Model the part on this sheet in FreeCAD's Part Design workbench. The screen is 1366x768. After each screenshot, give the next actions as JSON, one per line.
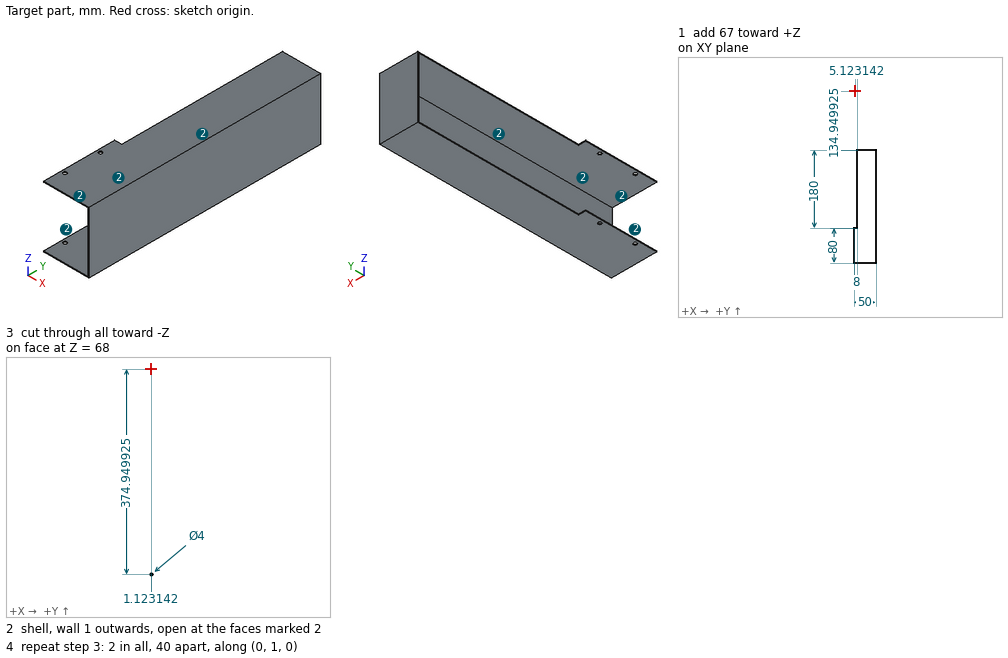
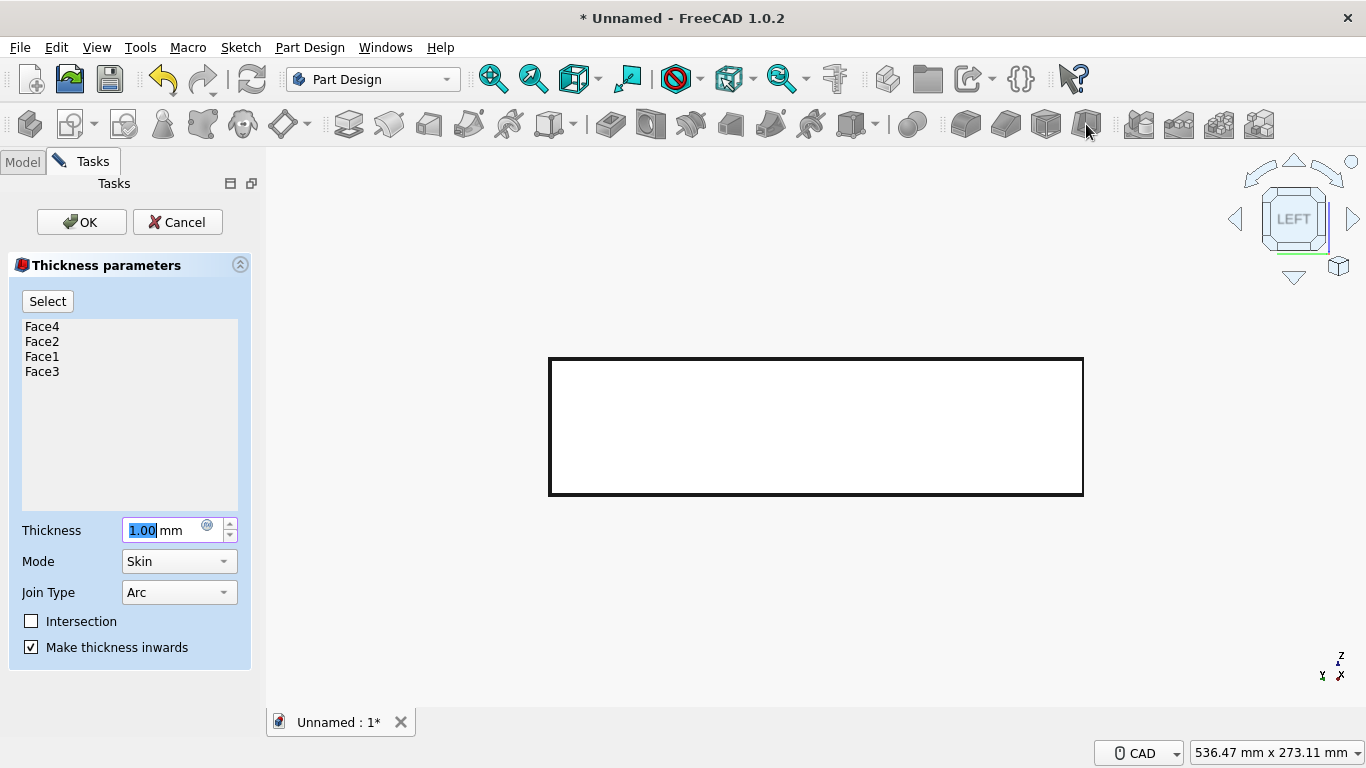
{"action": "type", "text": "1"}
{"action": "key", "text": "Tab"}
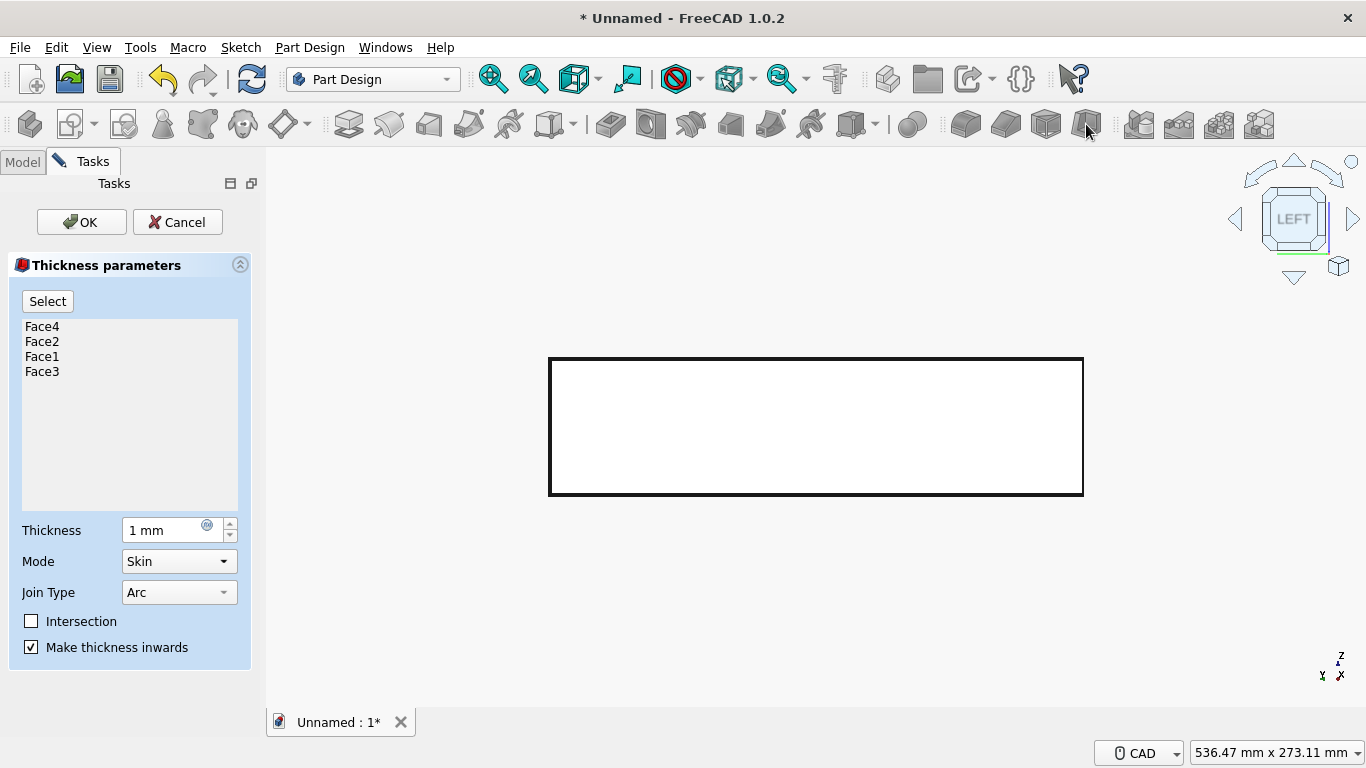
{"action": "left_click", "coordinate": [180, 592]}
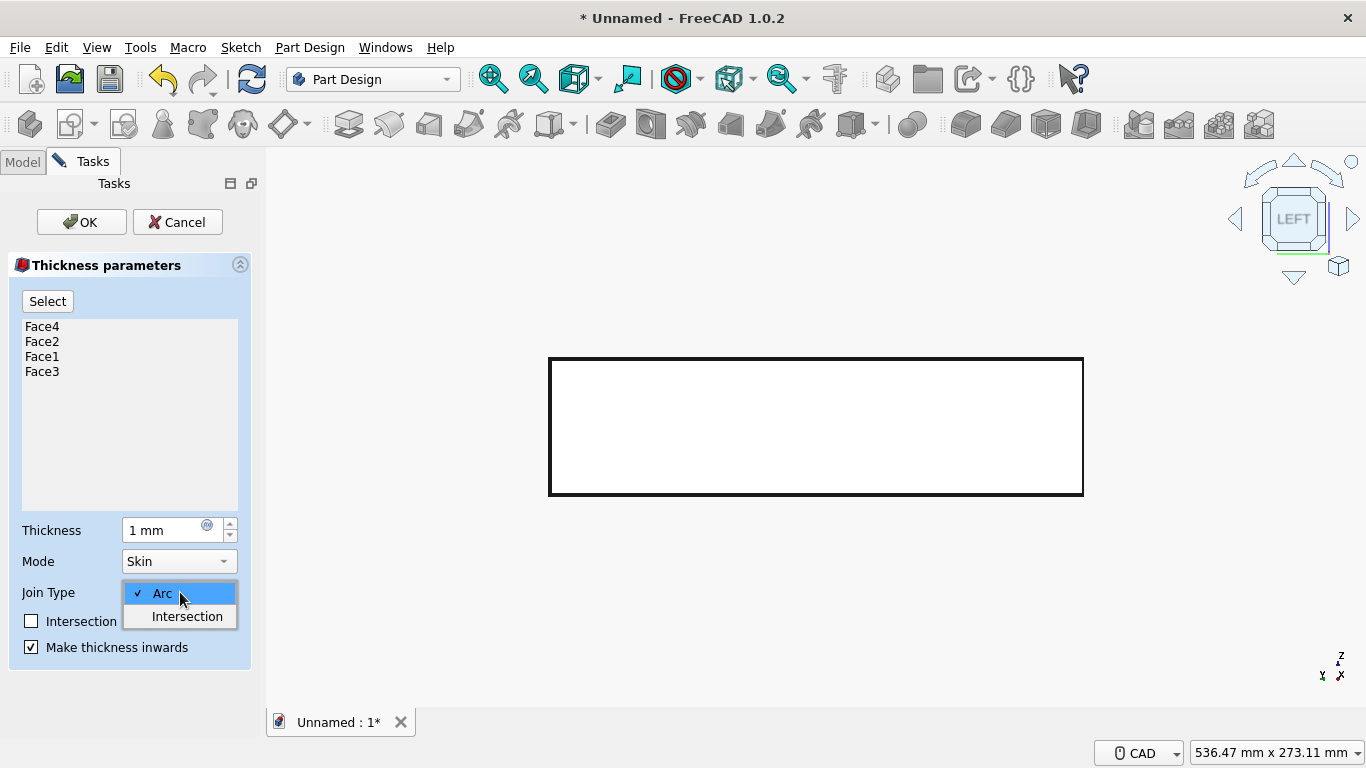
{"action": "left_click", "coordinate": [179, 616]}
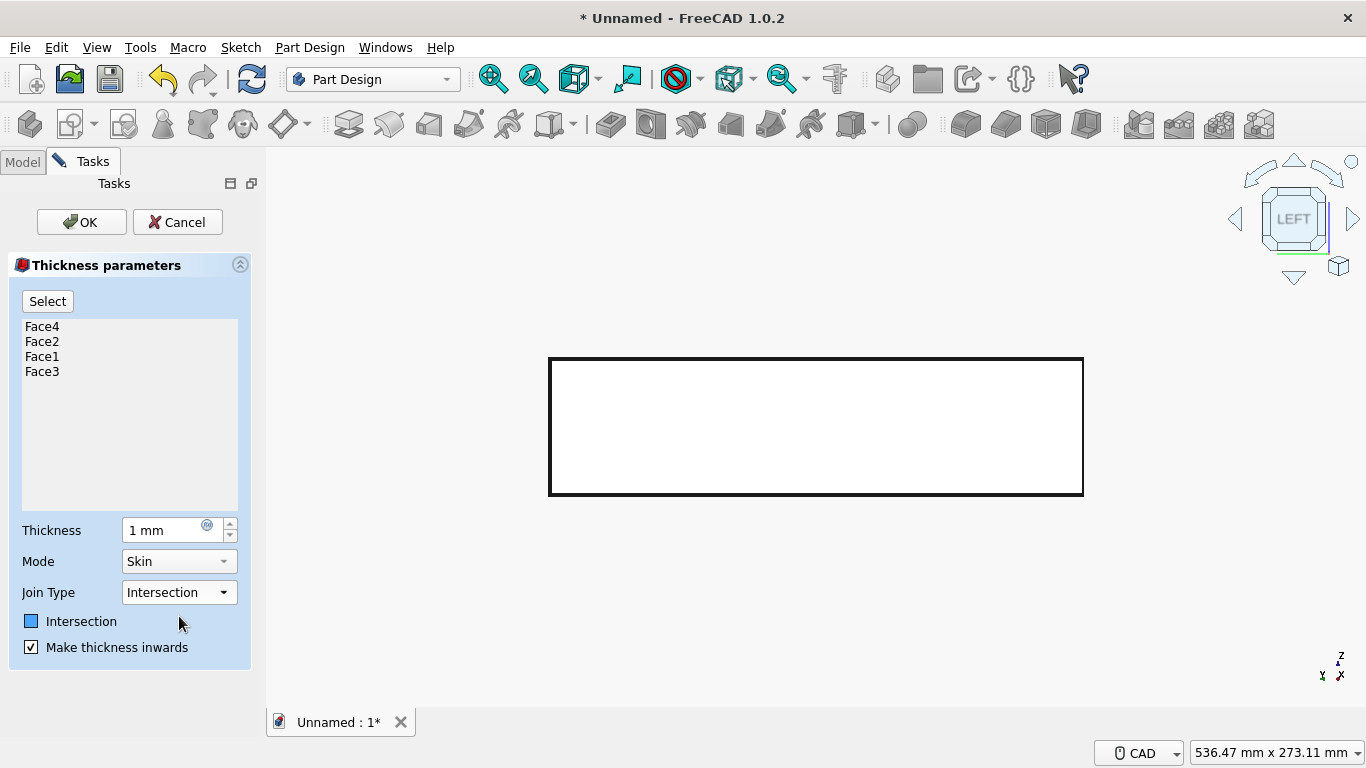
{"action": "left_click", "coordinate": [30, 647]}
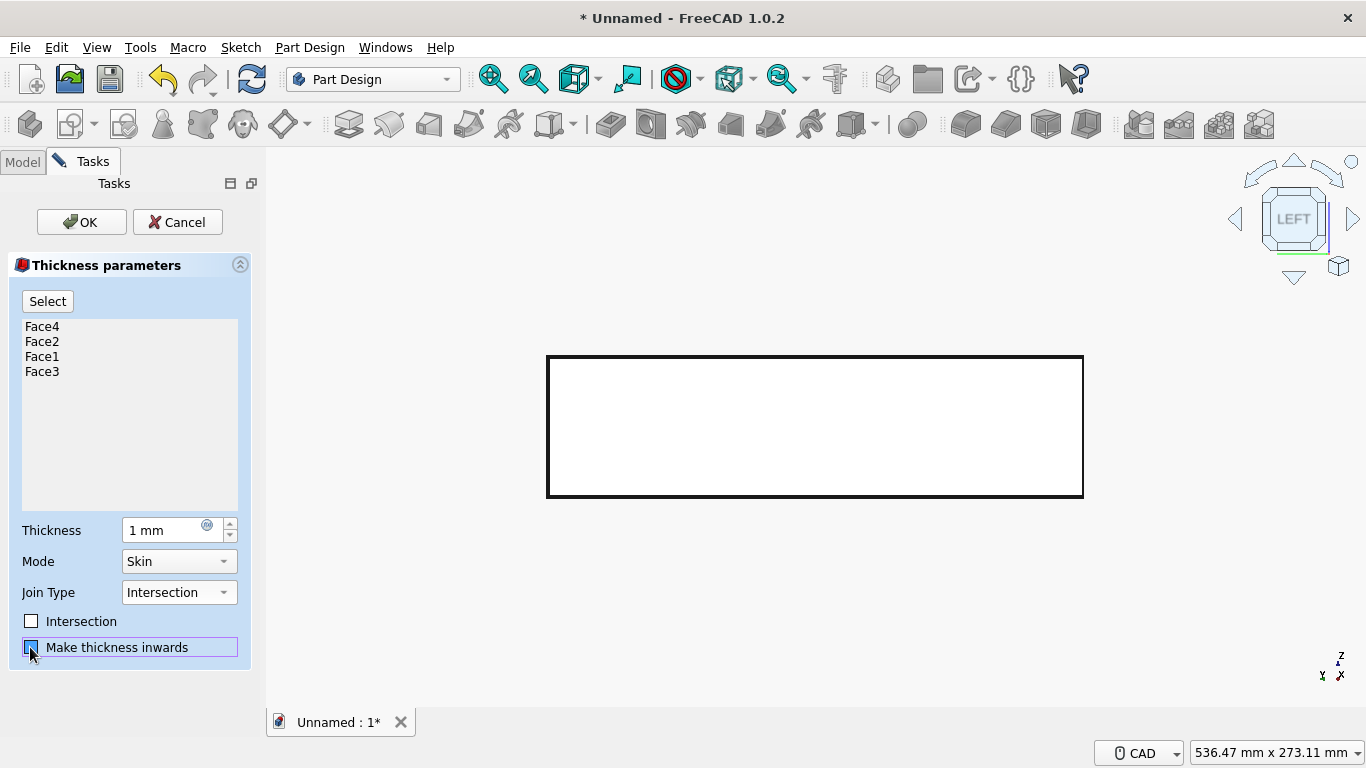
{"action": "left_click", "coordinate": [82, 222]}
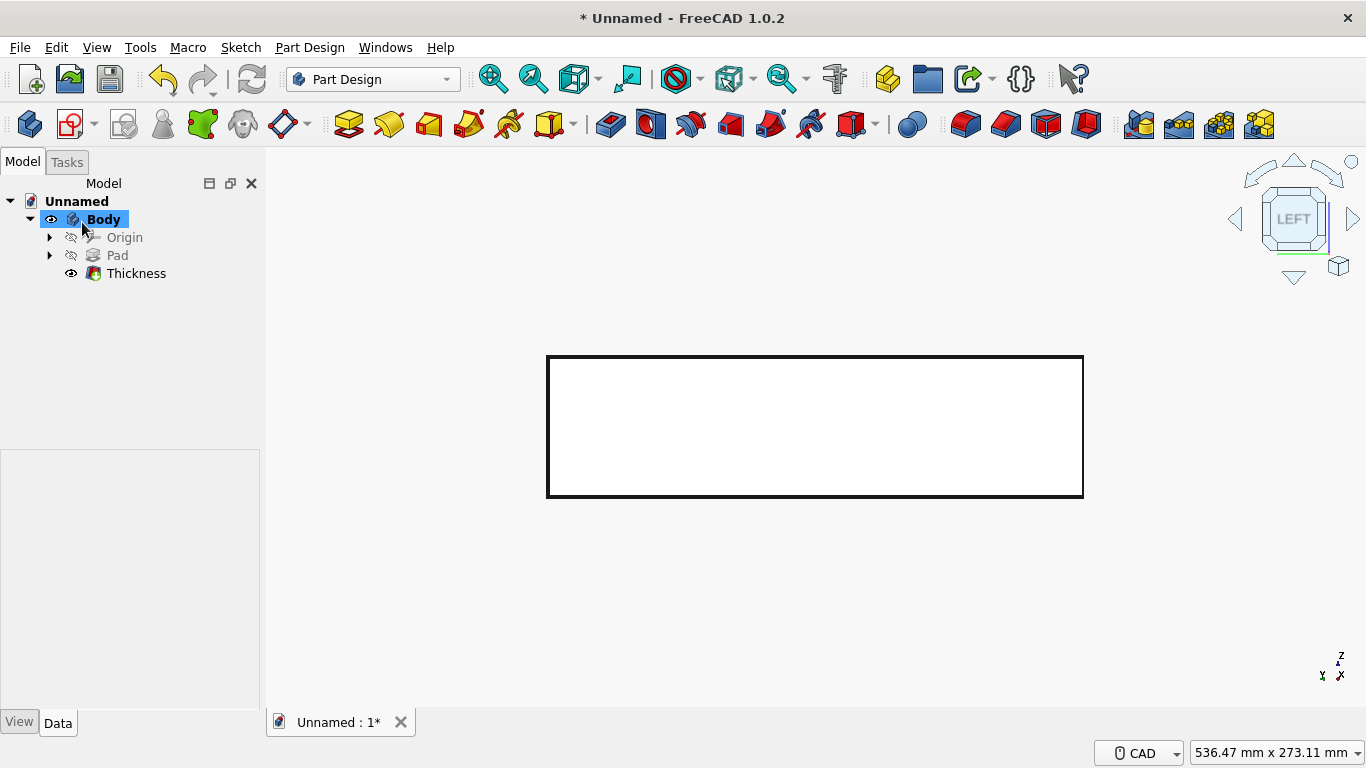
{"action": "key", "text": "0"}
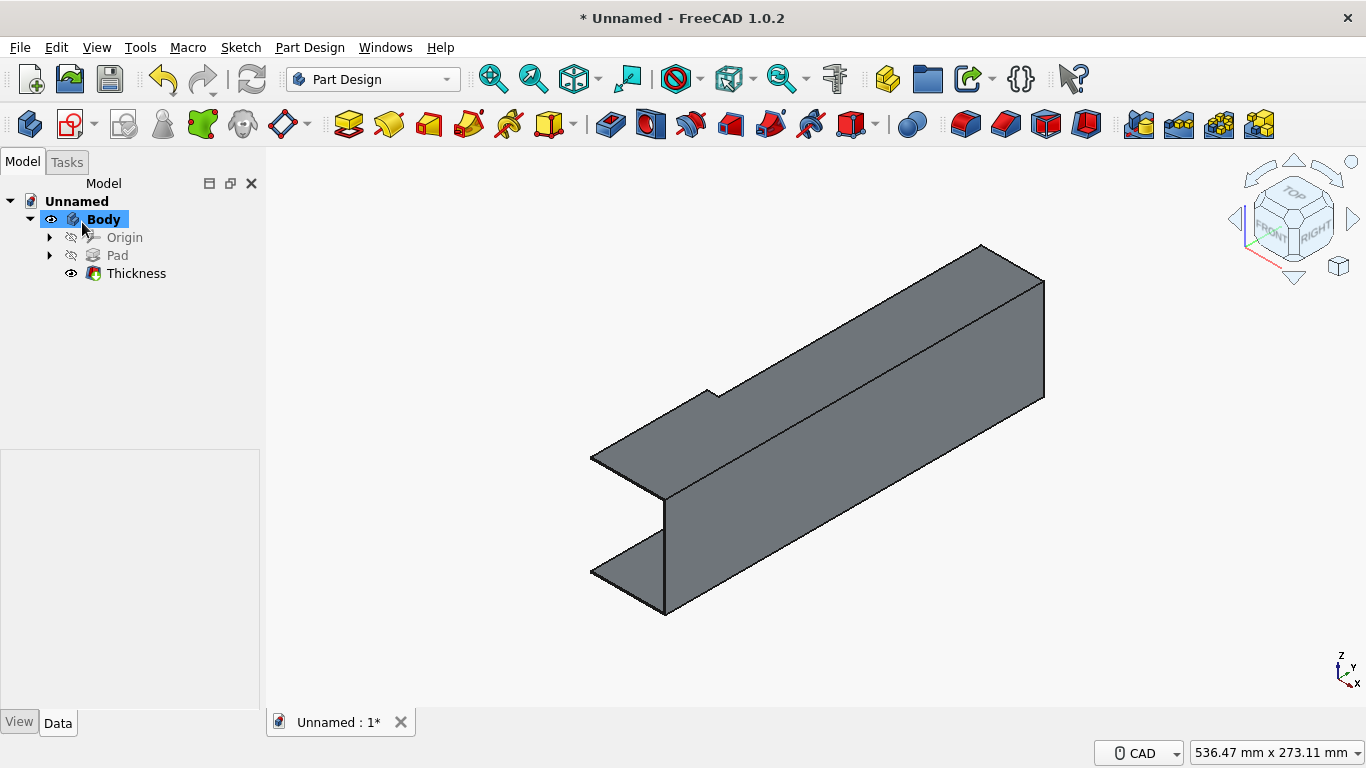
{"action": "left_click", "coordinate": [709, 431]}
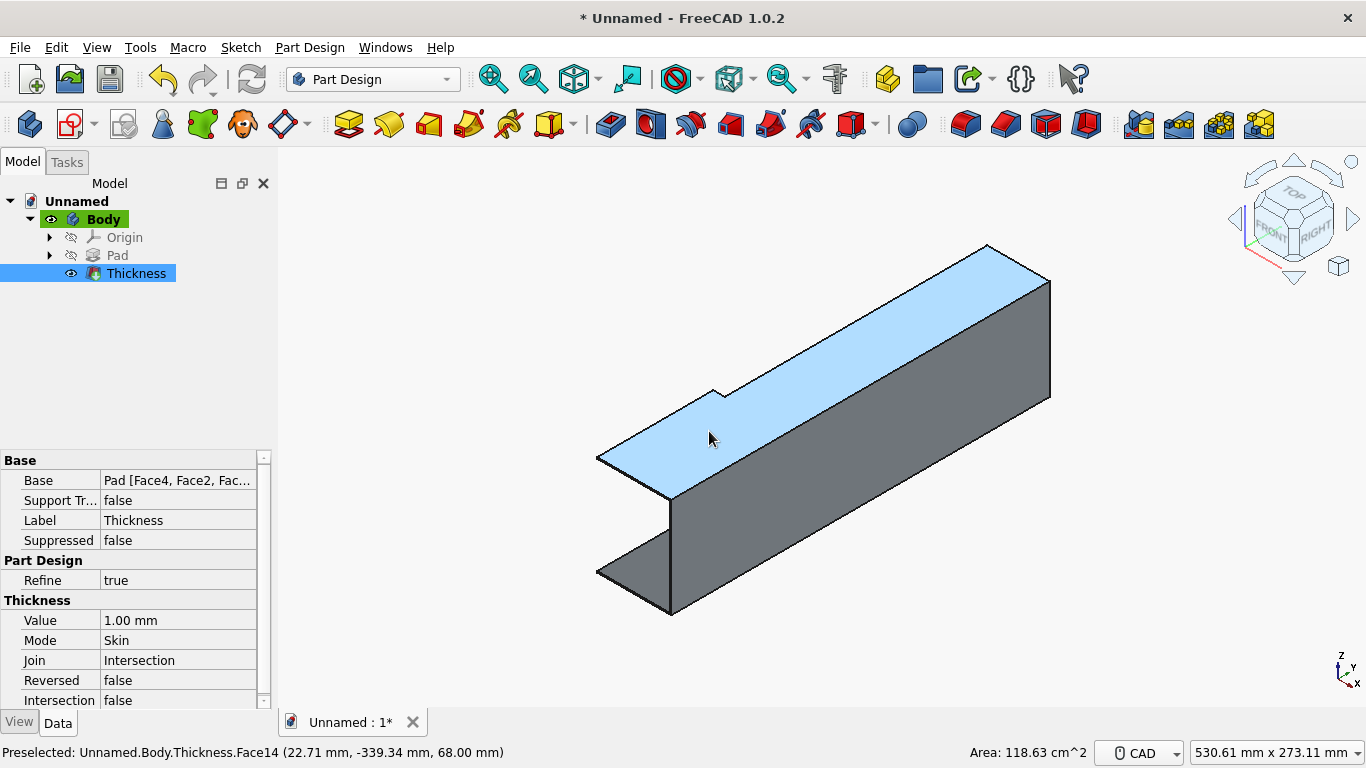
{"action": "left_click", "coordinate": [70, 124]}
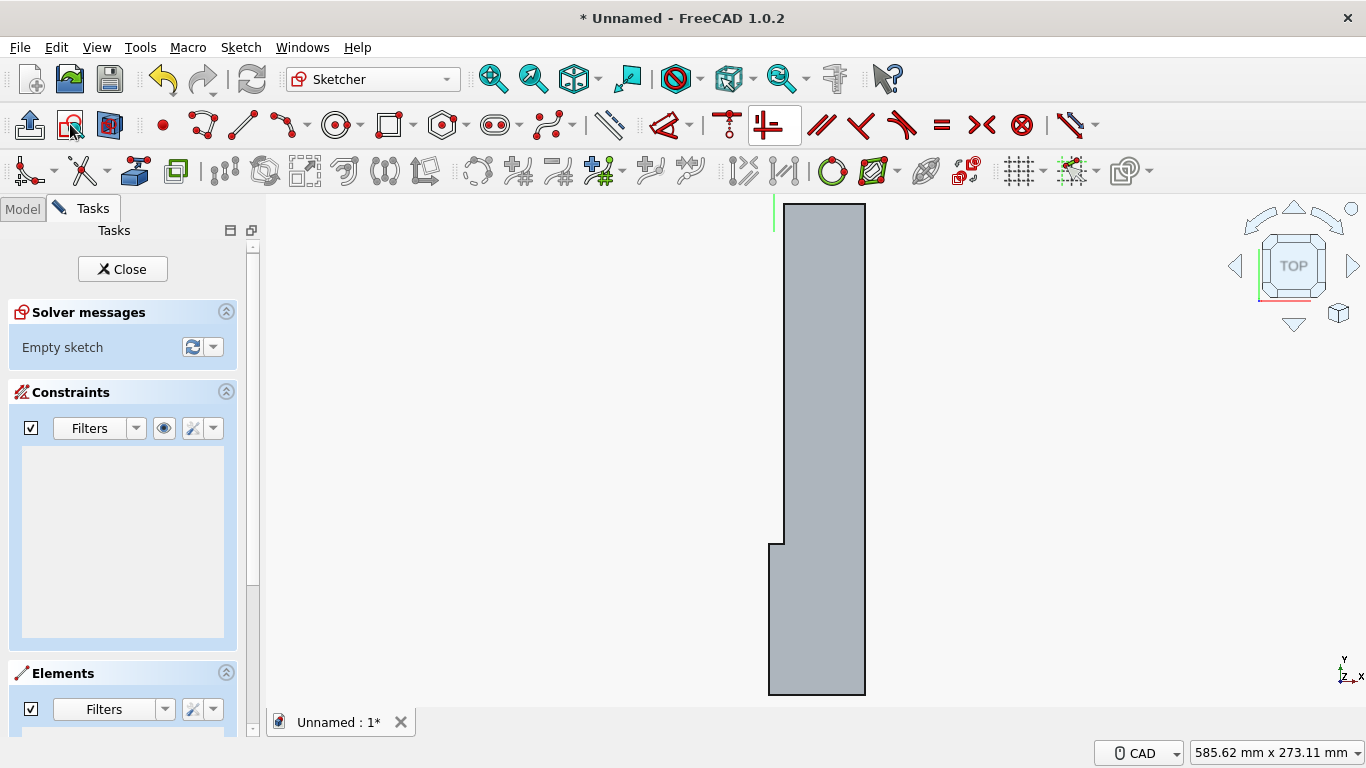
{"action": "scroll", "coordinate": [778, 668], "scroll_direction": "up", "scroll_amount": 15}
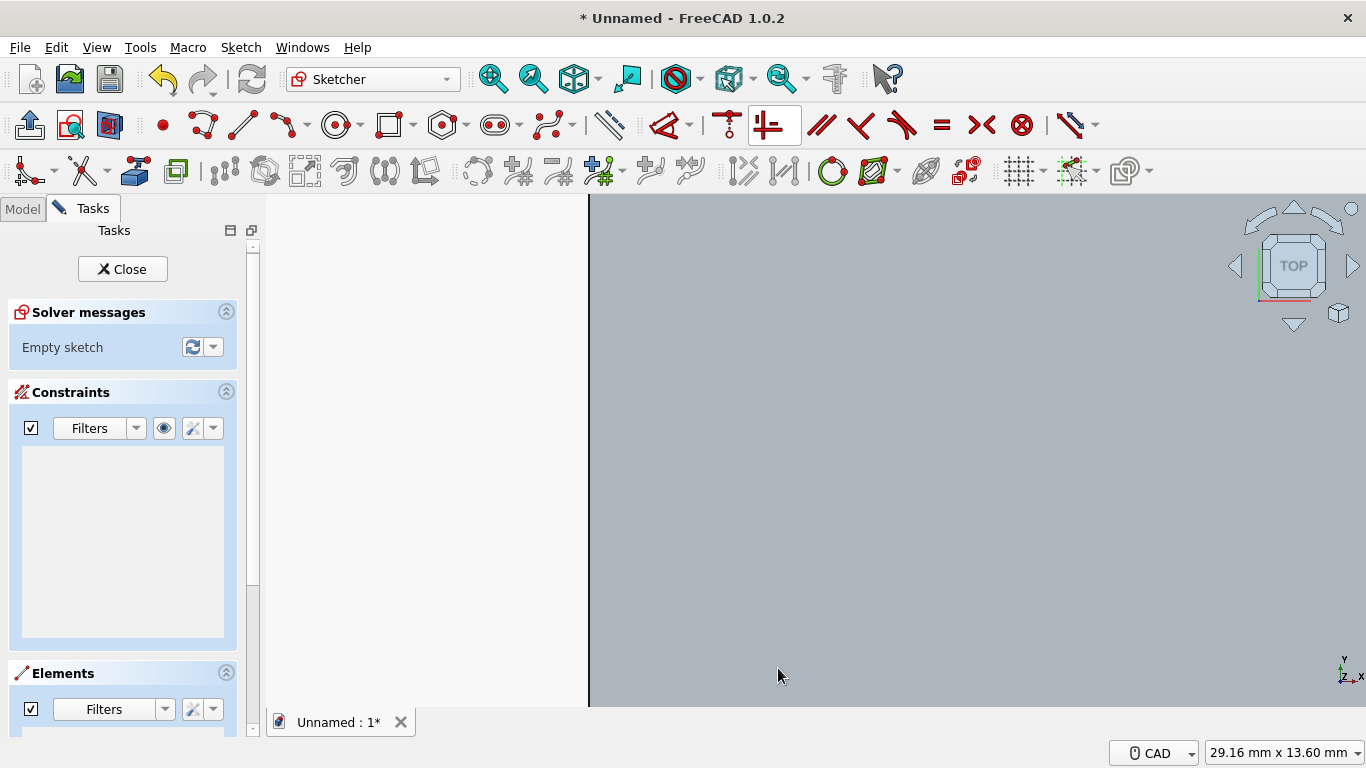
{"action": "scroll", "coordinate": [734, 417], "scroll_direction": "up", "scroll_amount": 4}